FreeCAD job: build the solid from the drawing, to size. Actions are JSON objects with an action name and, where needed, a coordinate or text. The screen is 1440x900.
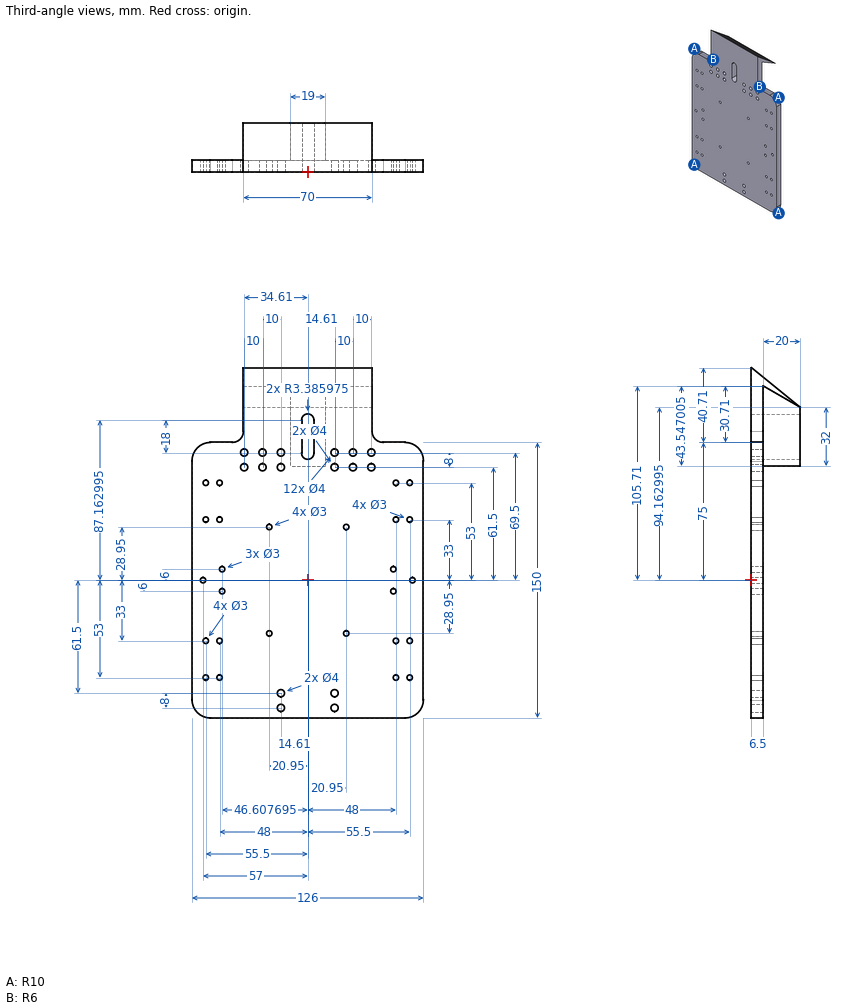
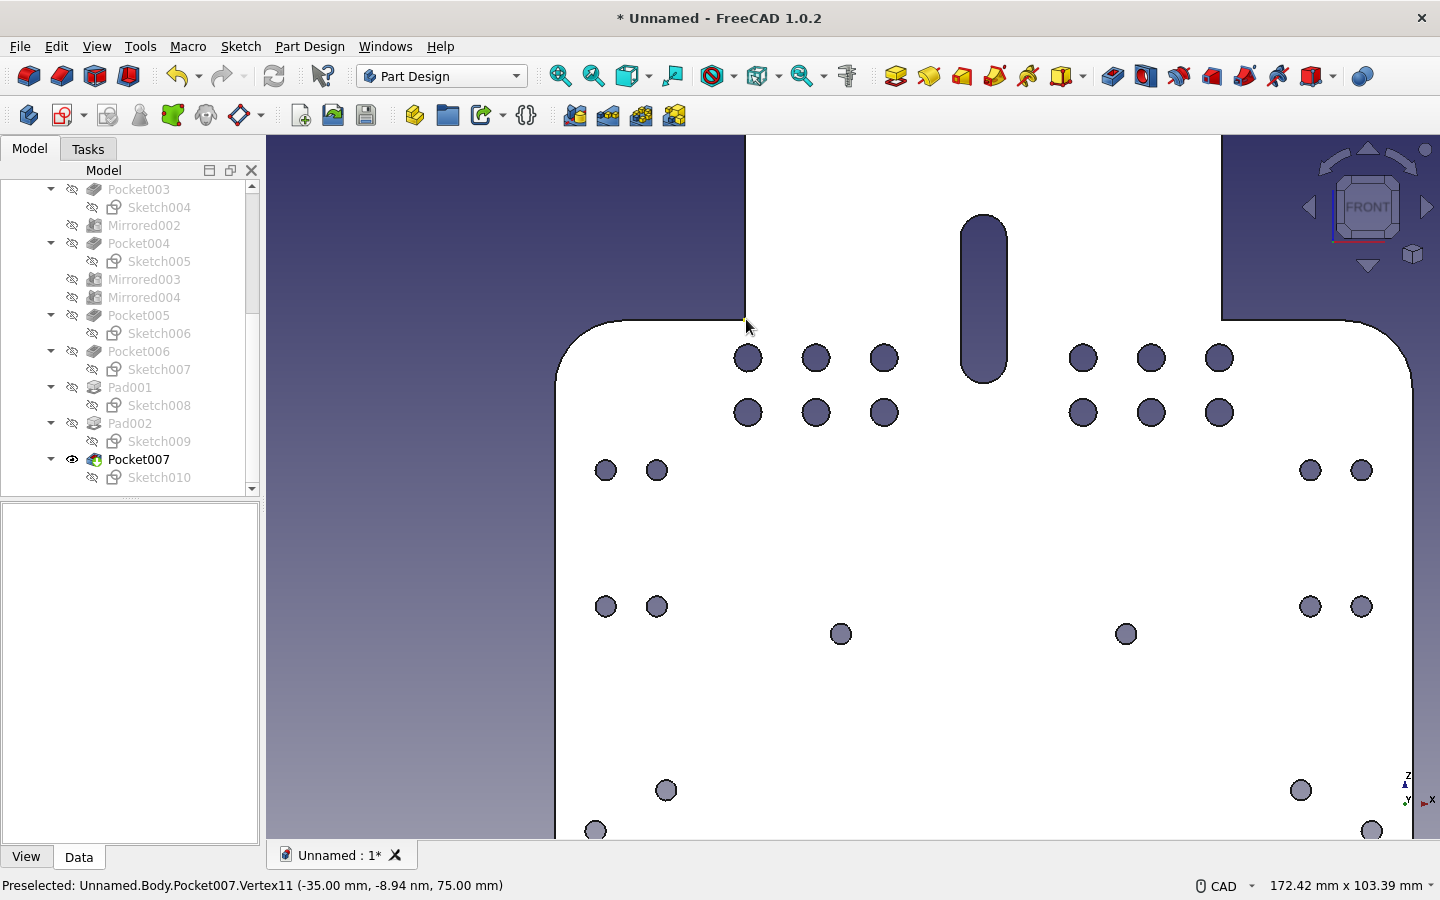
{"action": "key", "text": "v f"}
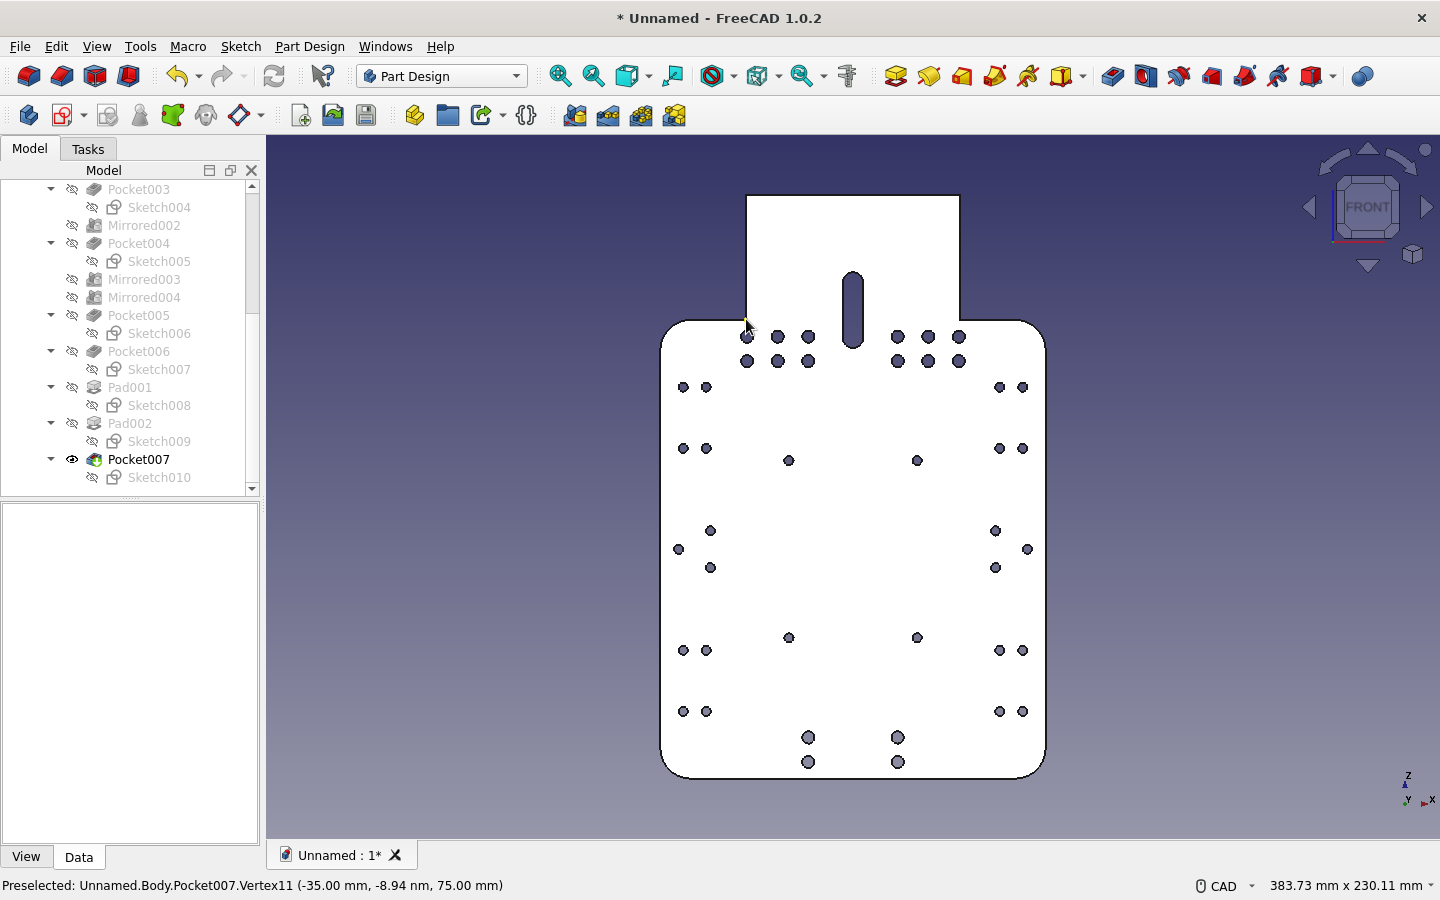
{"action": "key", "text": "3"}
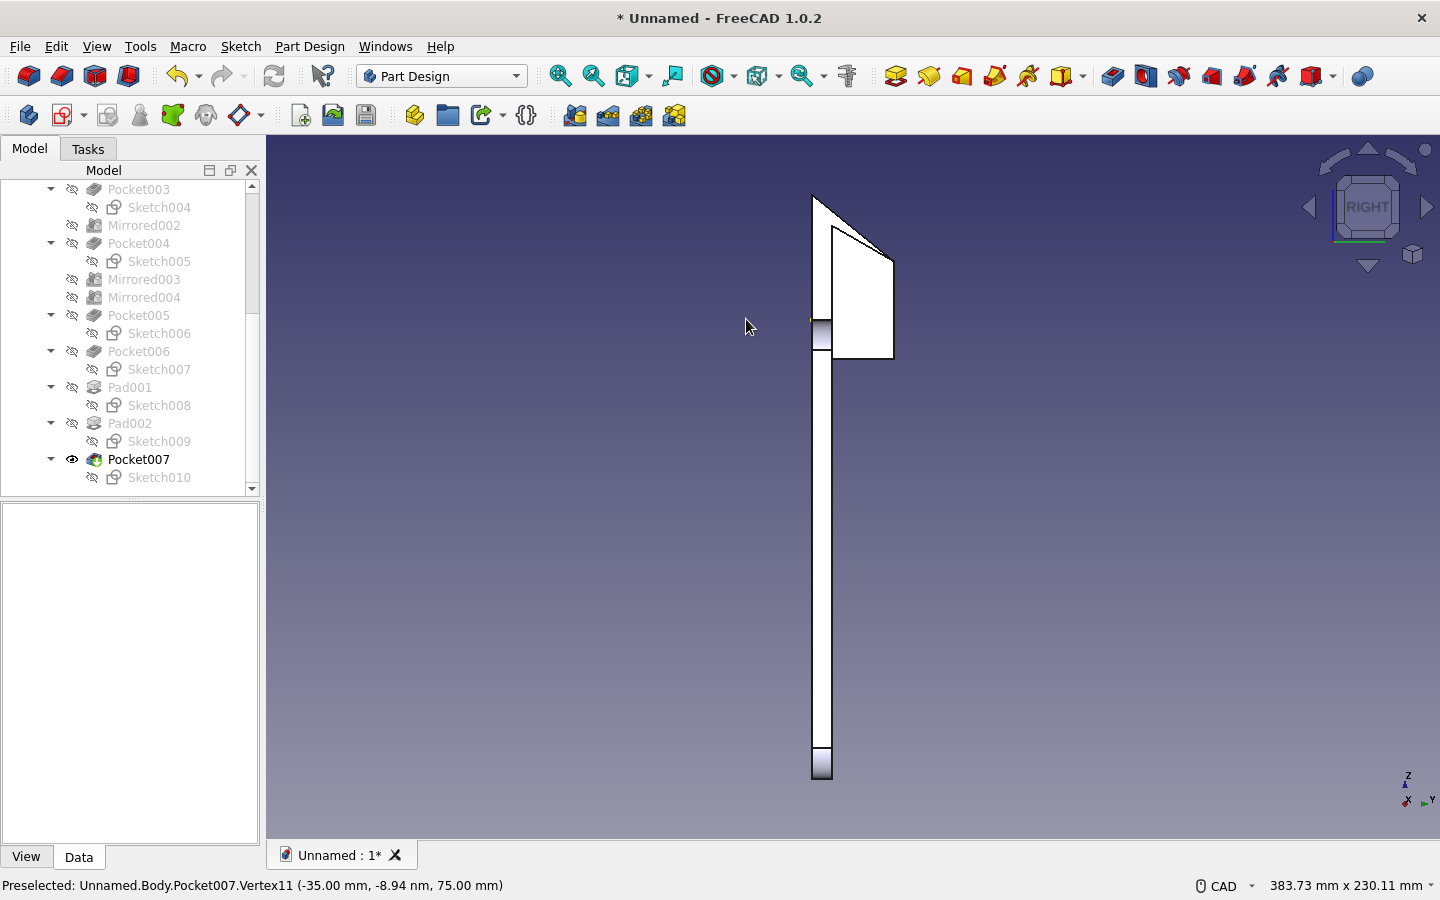
{"action": "scroll", "coordinate": [822, 319], "scroll_direction": "up", "scroll_amount": 4}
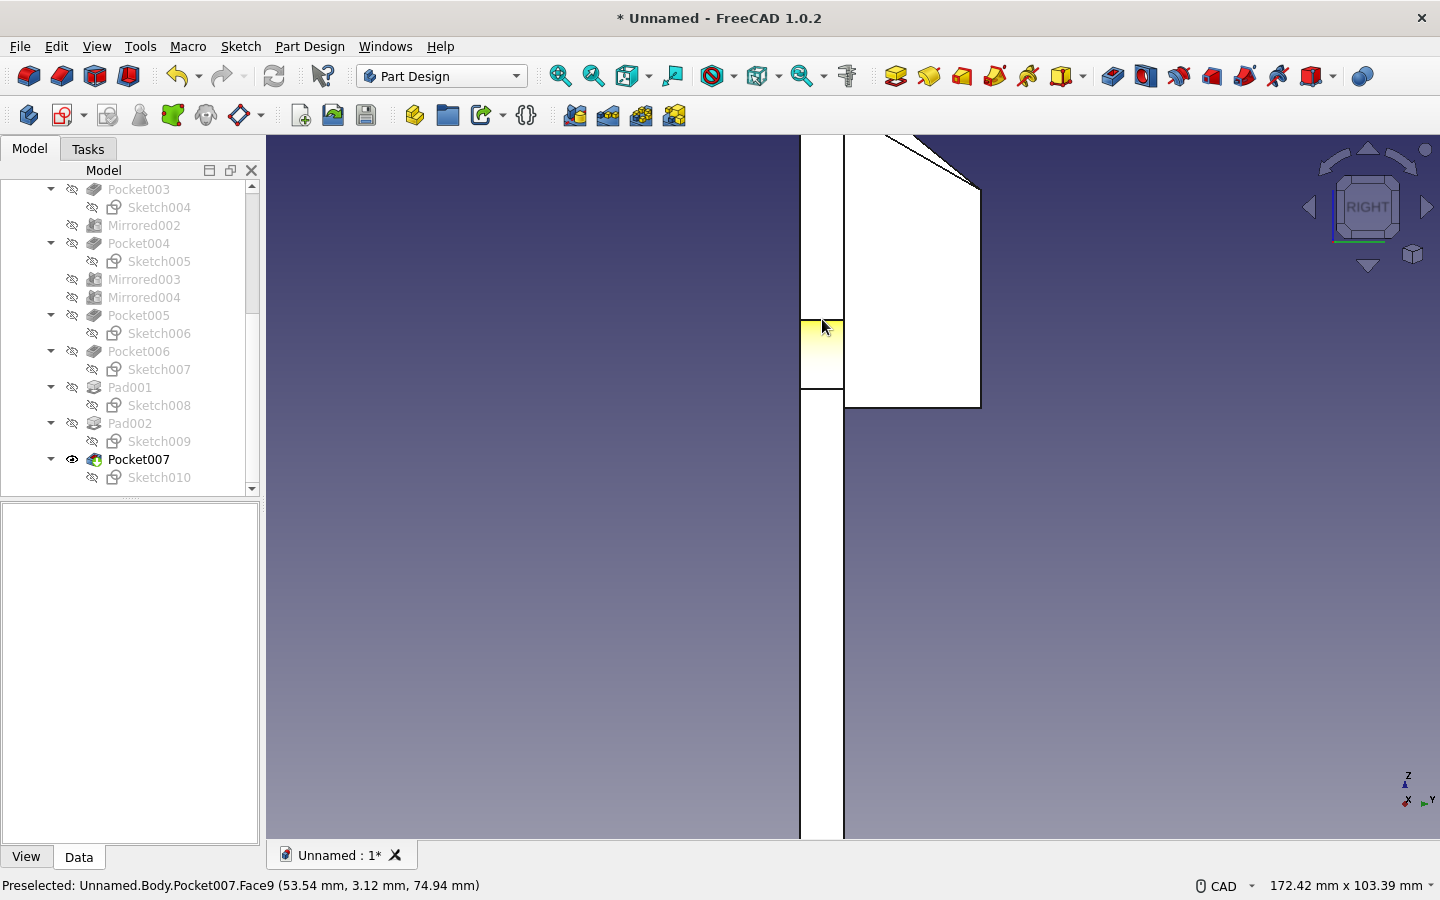
{"action": "left_click", "coordinate": [561, 76]}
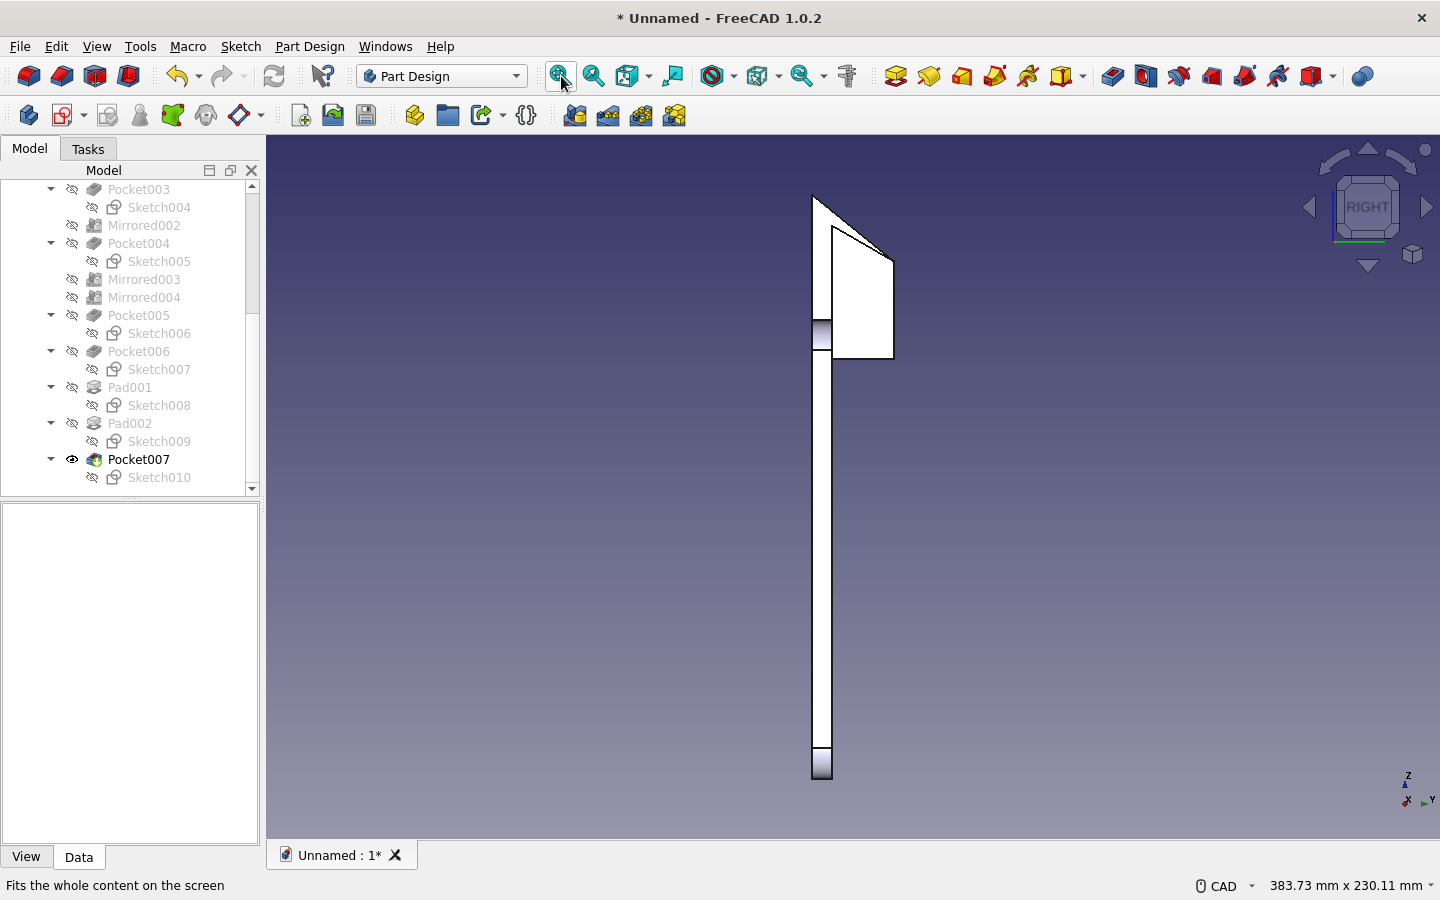
{"action": "key", "text": "5"}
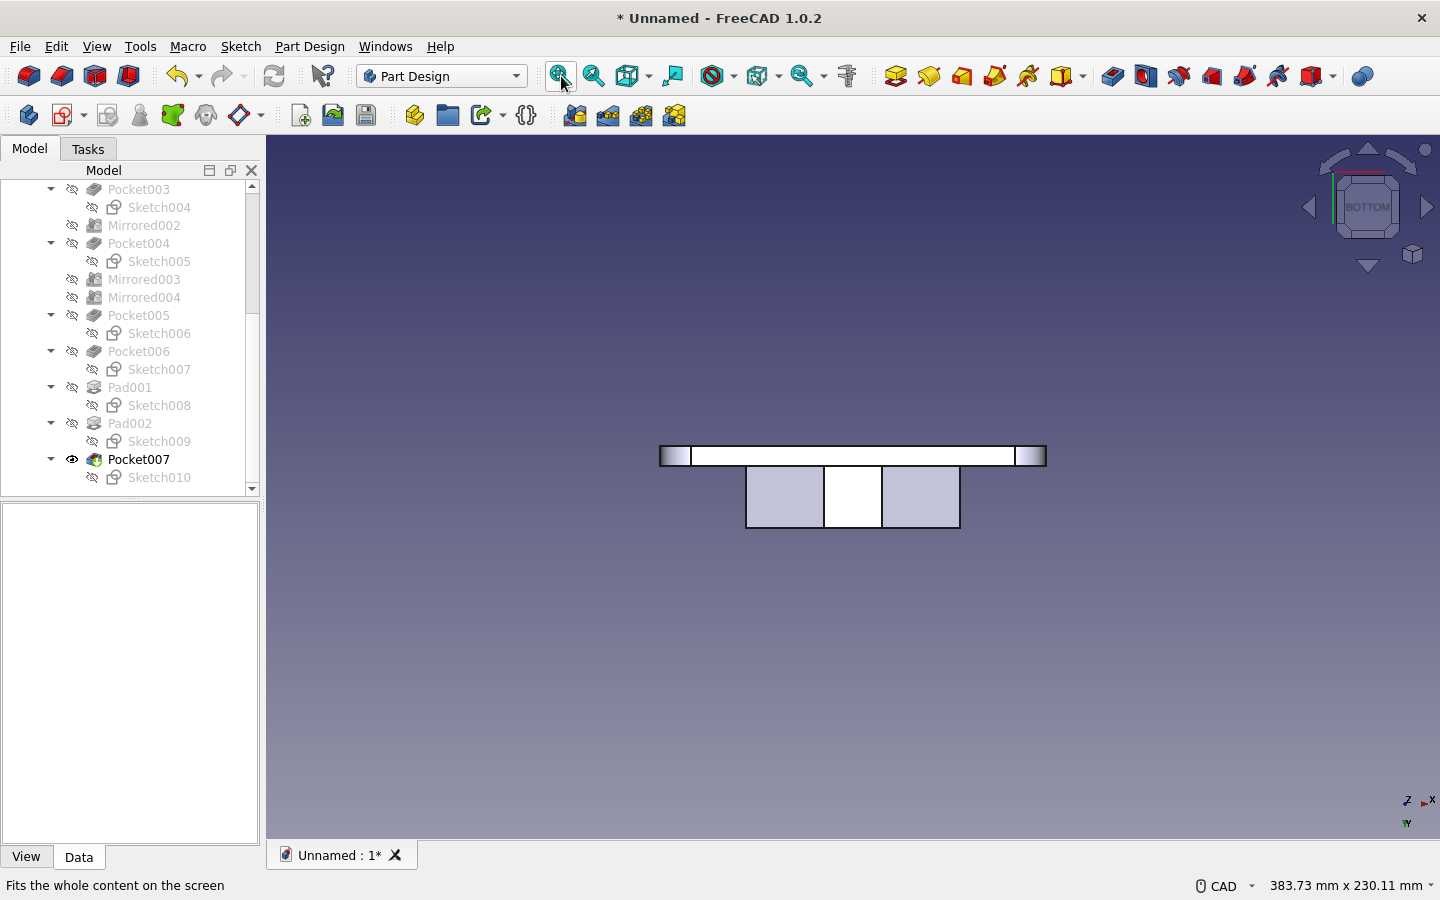
{"action": "key", "text": "v f"}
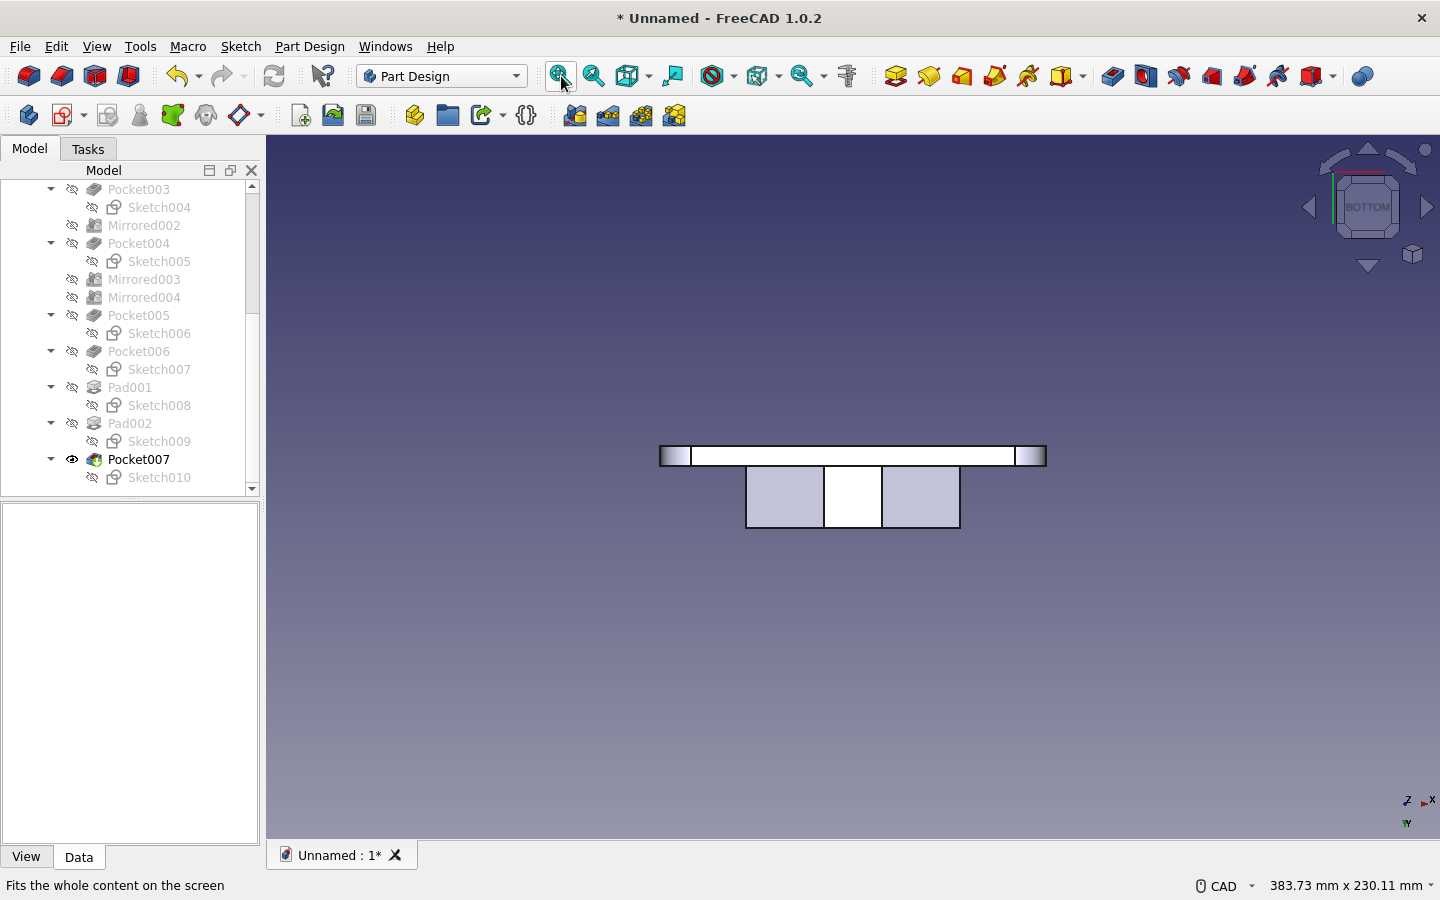
{"action": "scroll", "coordinate": [746, 455], "scroll_direction": "up", "scroll_amount": 4}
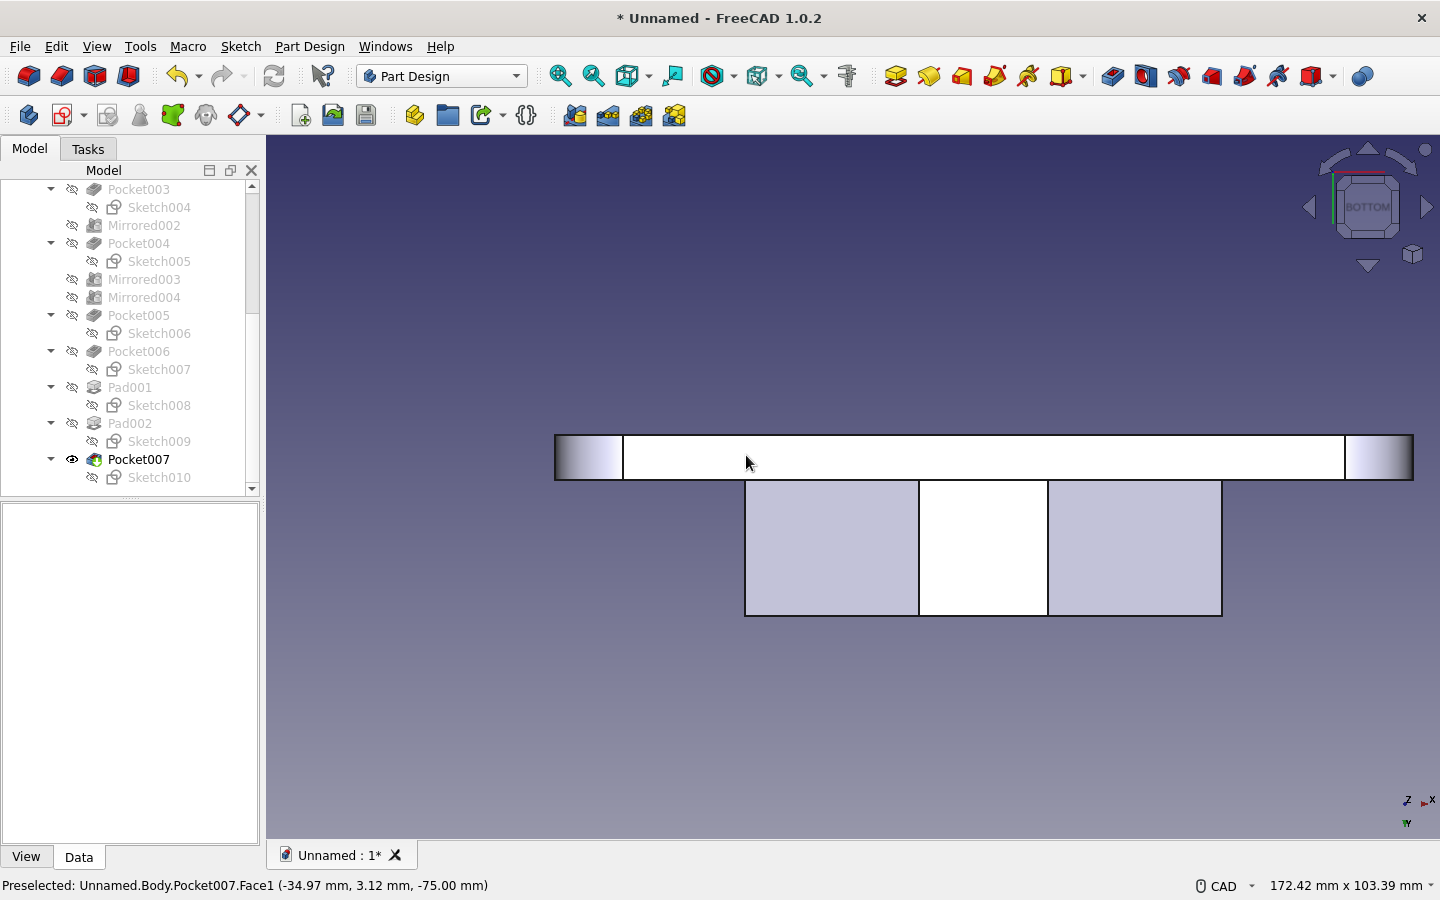
{"action": "key", "text": "v f"}